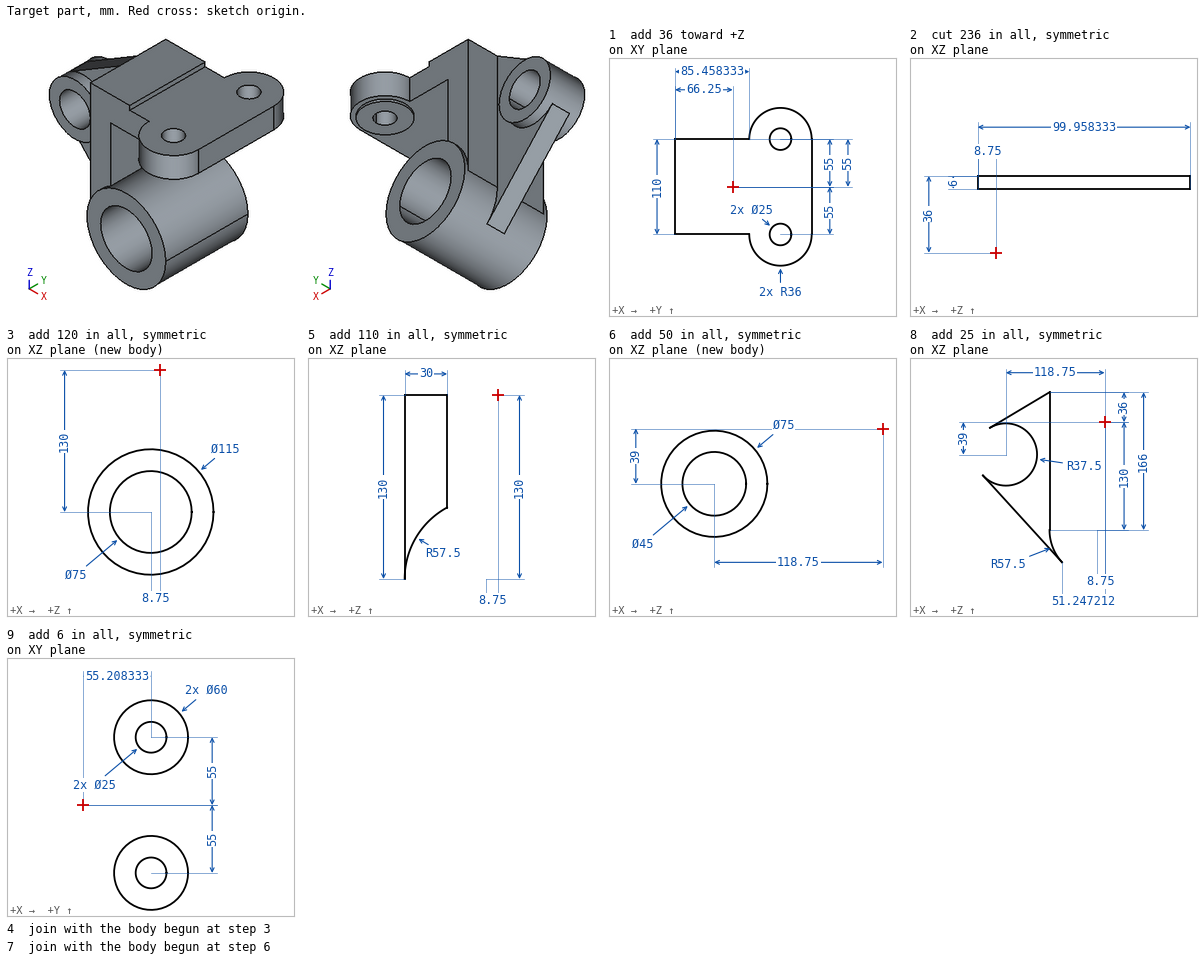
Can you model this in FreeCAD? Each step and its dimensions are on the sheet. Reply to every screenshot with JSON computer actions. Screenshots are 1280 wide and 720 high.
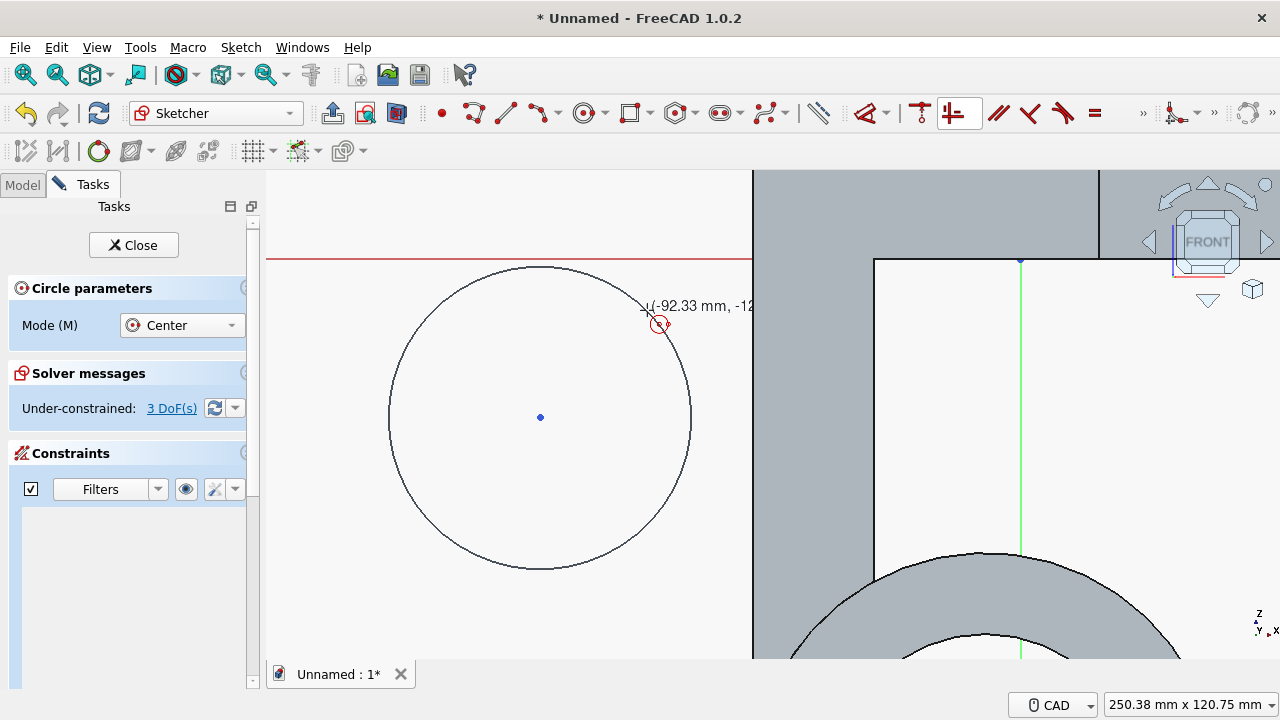
{"action": "left_click", "coordinate": [540, 418]}
{"action": "left_click", "coordinate": [604, 353]}
{"action": "key", "text": "Escape"}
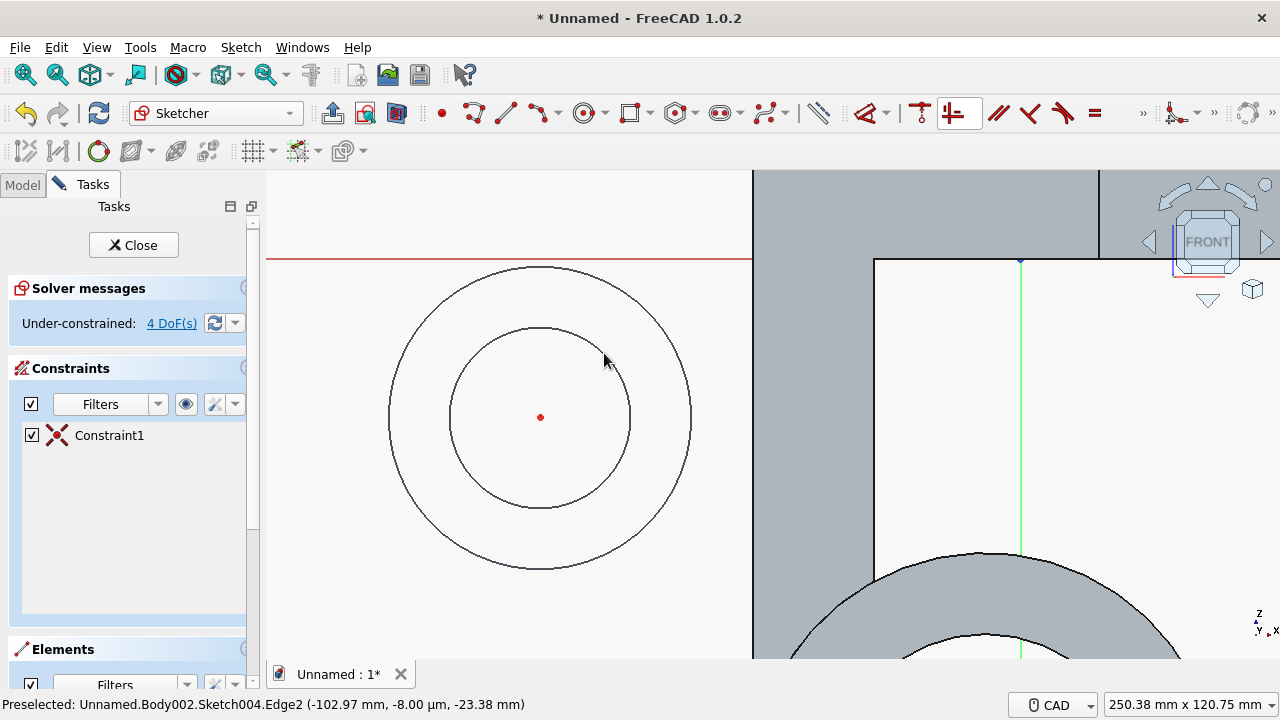
{"action": "left_click", "coordinate": [866, 114]}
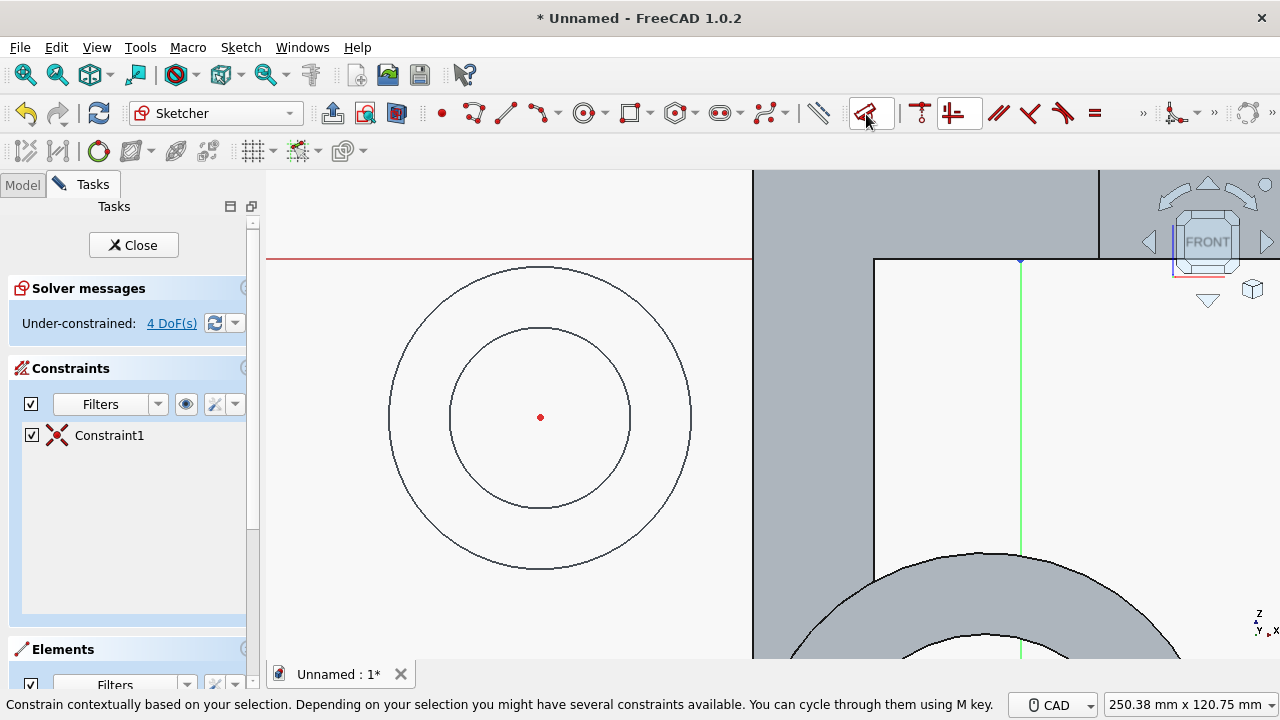
{"action": "left_click", "coordinate": [647, 311]}
{"action": "left_click", "coordinate": [670, 288]}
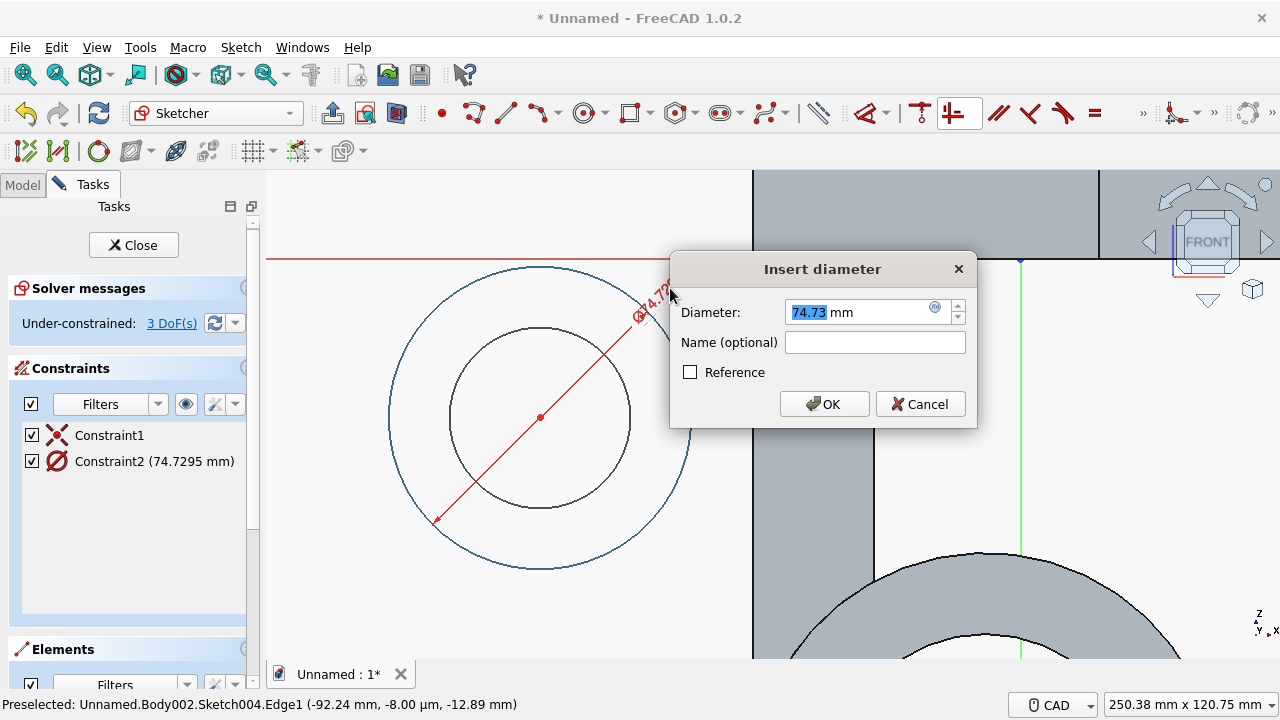
{"action": "type", "text": "75"}
{"action": "key", "text": "Return"}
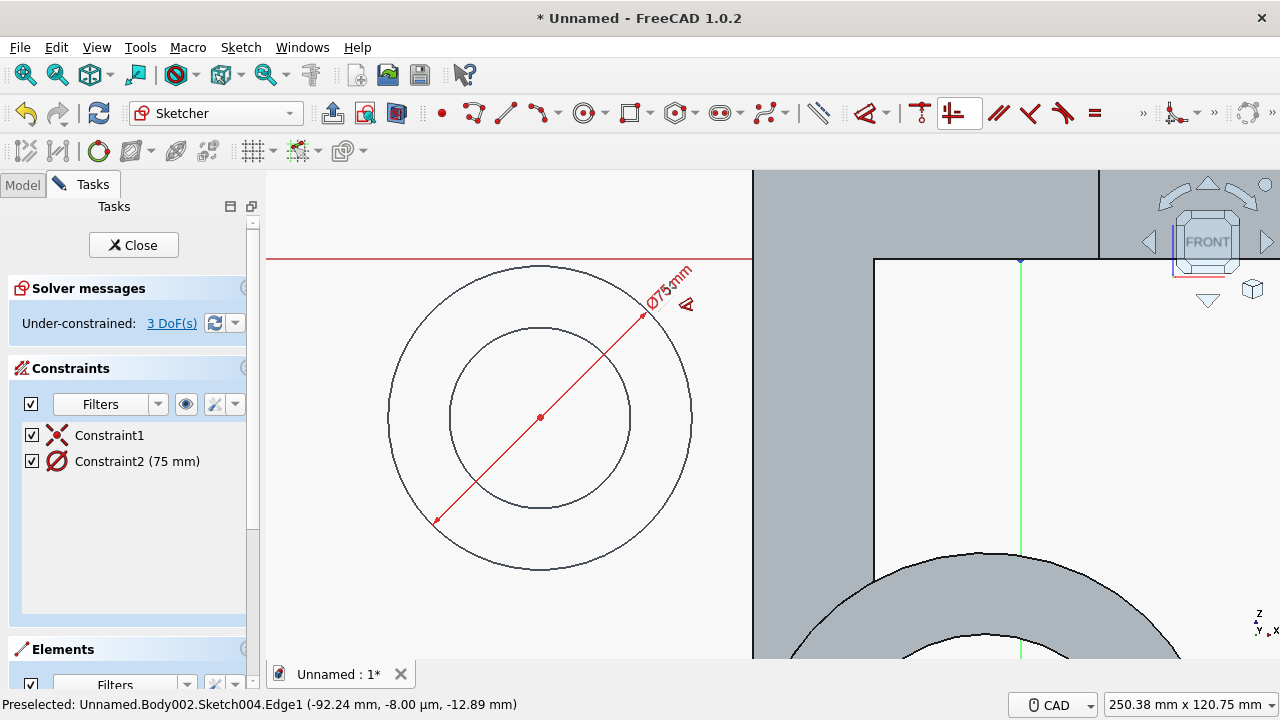
{"action": "left_click", "coordinate": [604, 354]}
{"action": "left_click", "coordinate": [627, 331]}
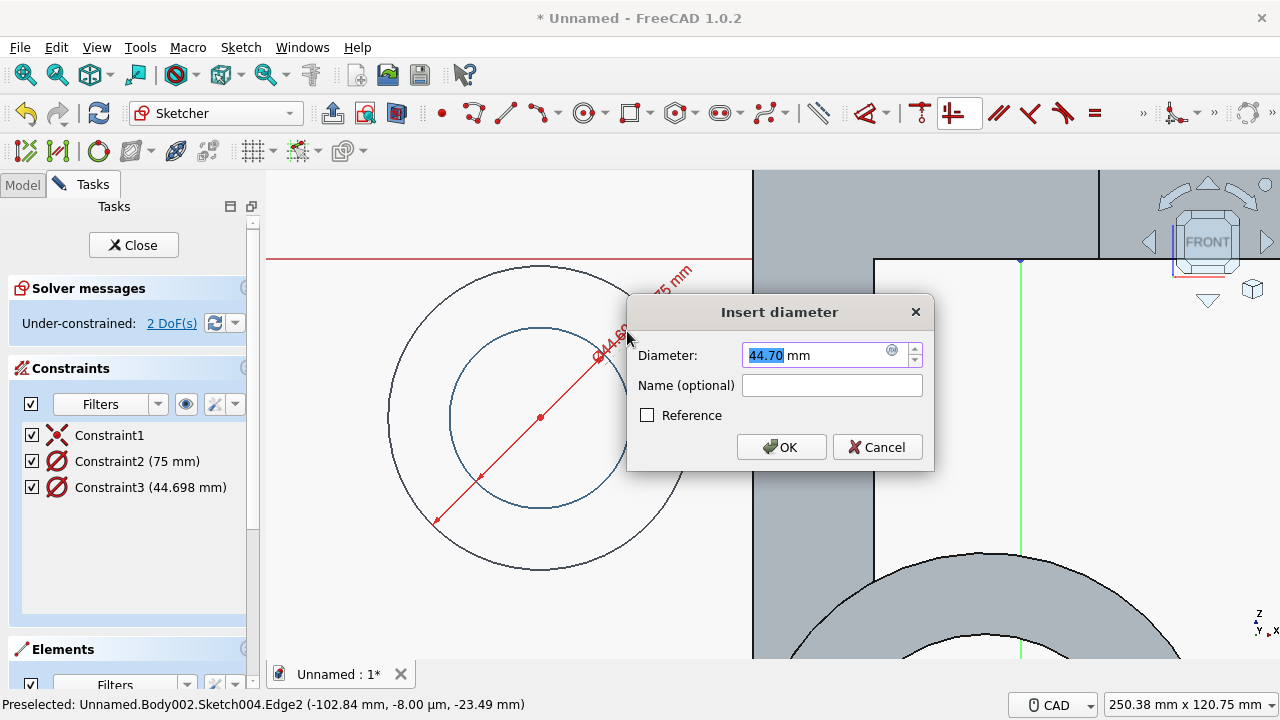
{"action": "type", "text": "45"}
{"action": "key", "text": "Return"}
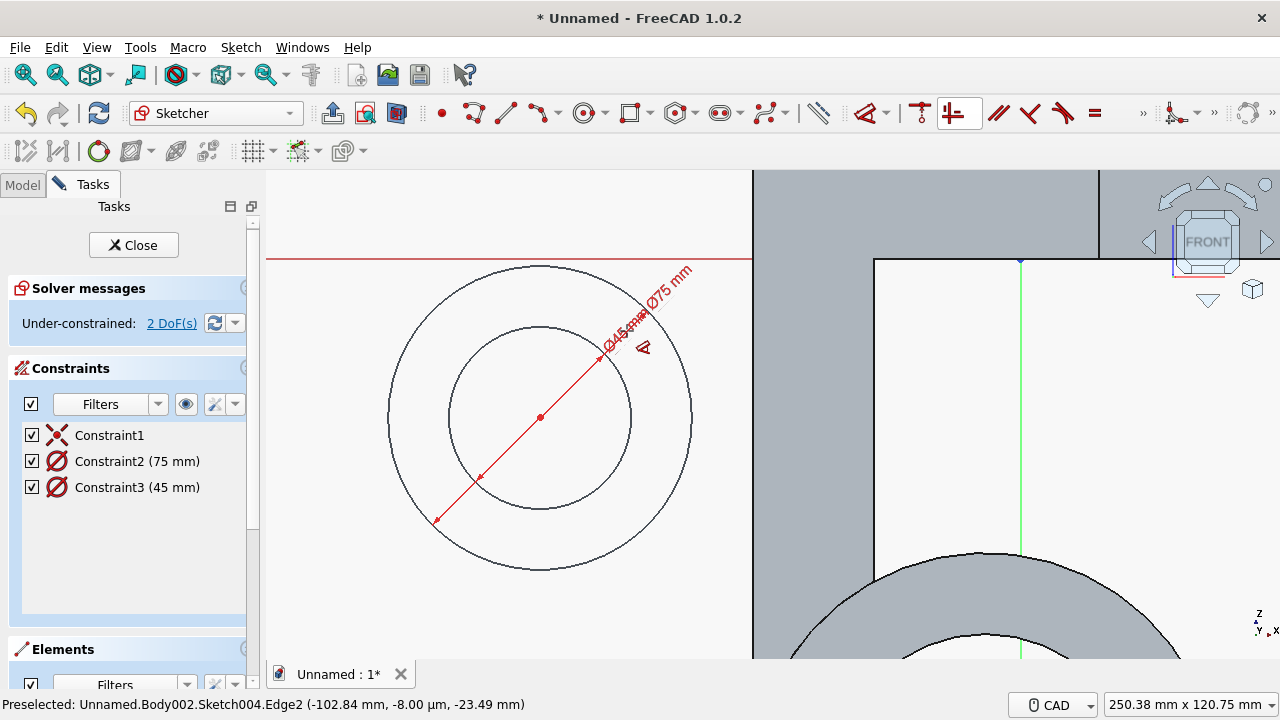
{"action": "left_click", "coordinate": [540, 418]}
{"action": "left_click", "coordinate": [1055, 339]}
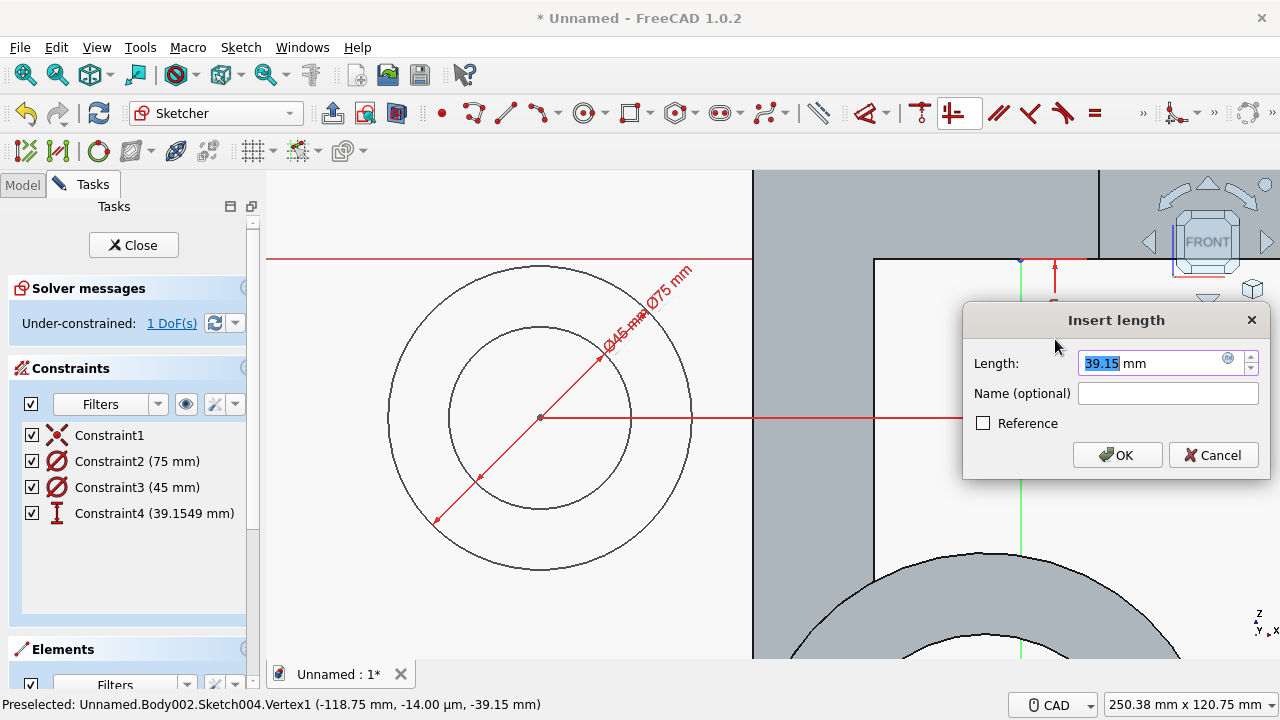
{"action": "type", "text": "39"}
{"action": "key", "text": "Return"}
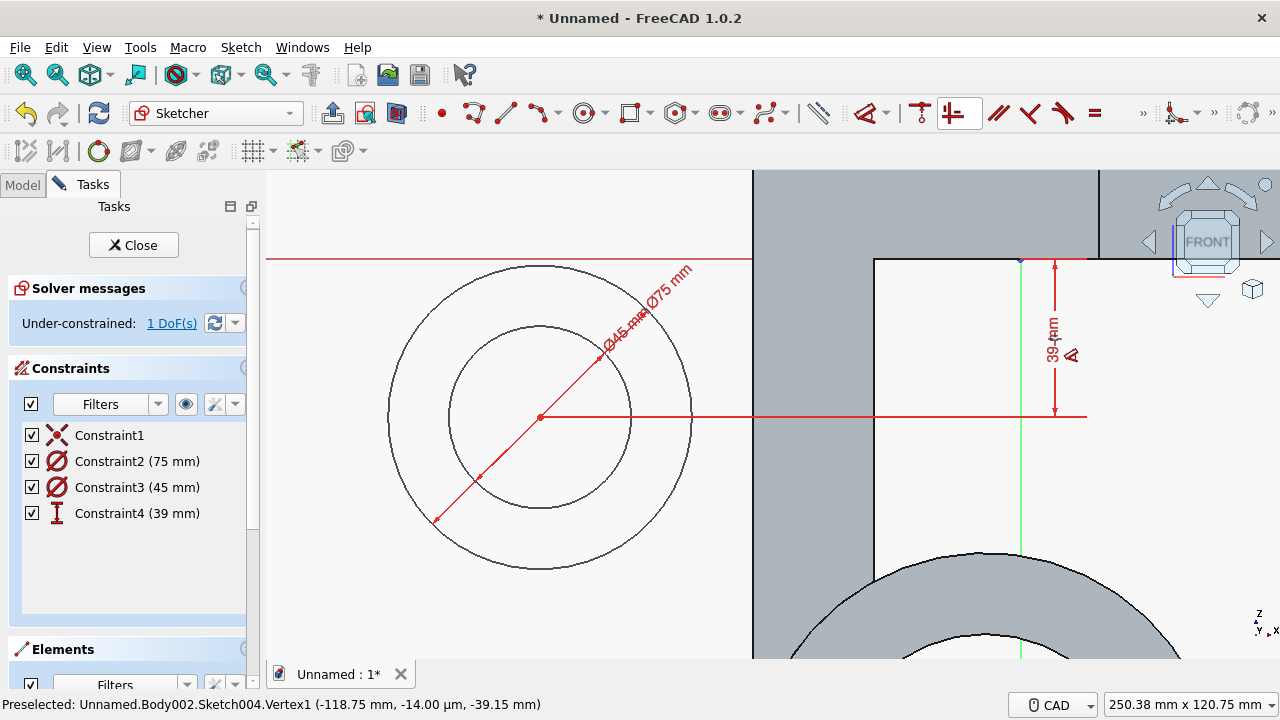
{"action": "left_click", "coordinate": [540, 417]}
{"action": "left_click", "coordinate": [780, 225]}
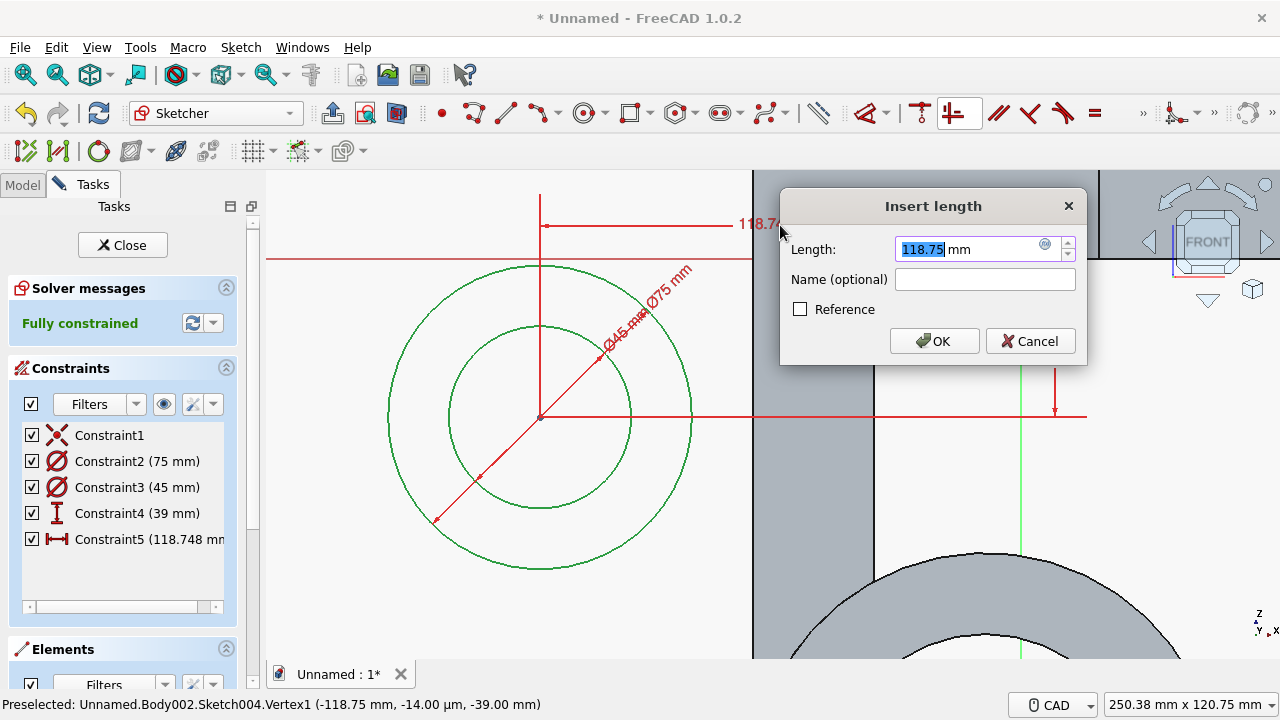
{"action": "type", "text": "118.75"}
{"action": "key", "text": "Return"}
{"action": "key", "text": "Escape"}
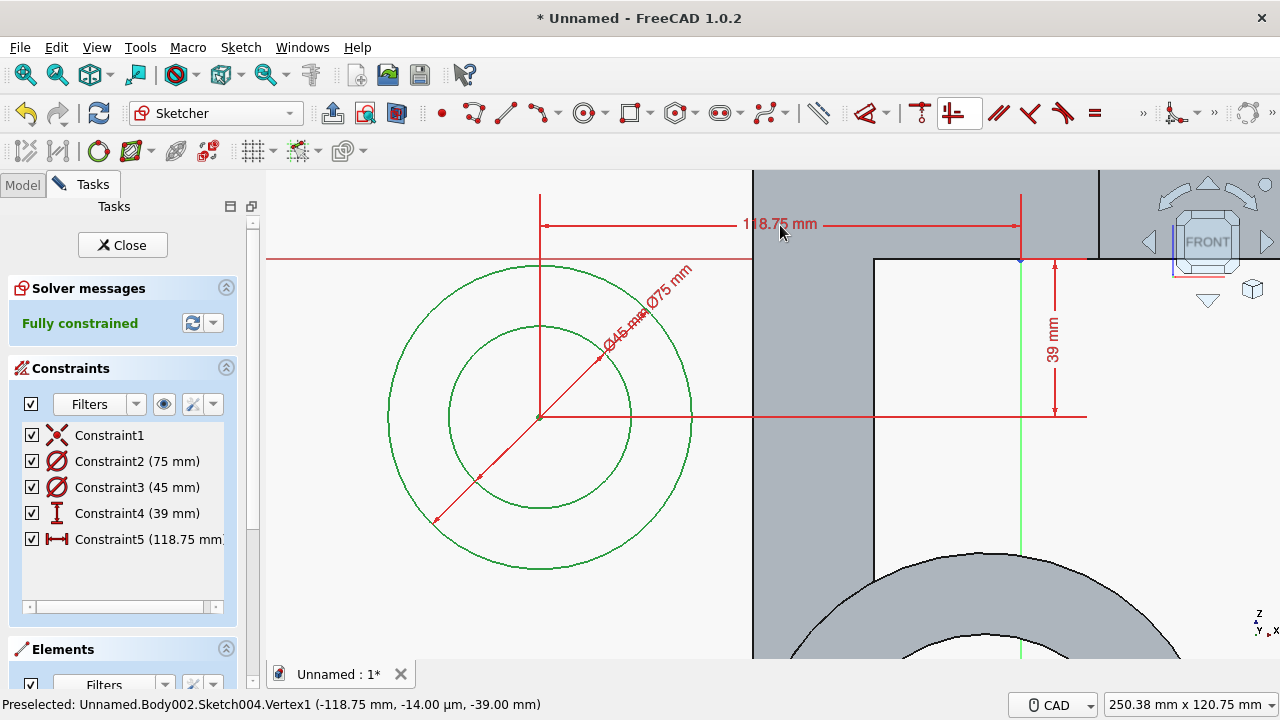
{"action": "left_click", "coordinate": [123, 245]}